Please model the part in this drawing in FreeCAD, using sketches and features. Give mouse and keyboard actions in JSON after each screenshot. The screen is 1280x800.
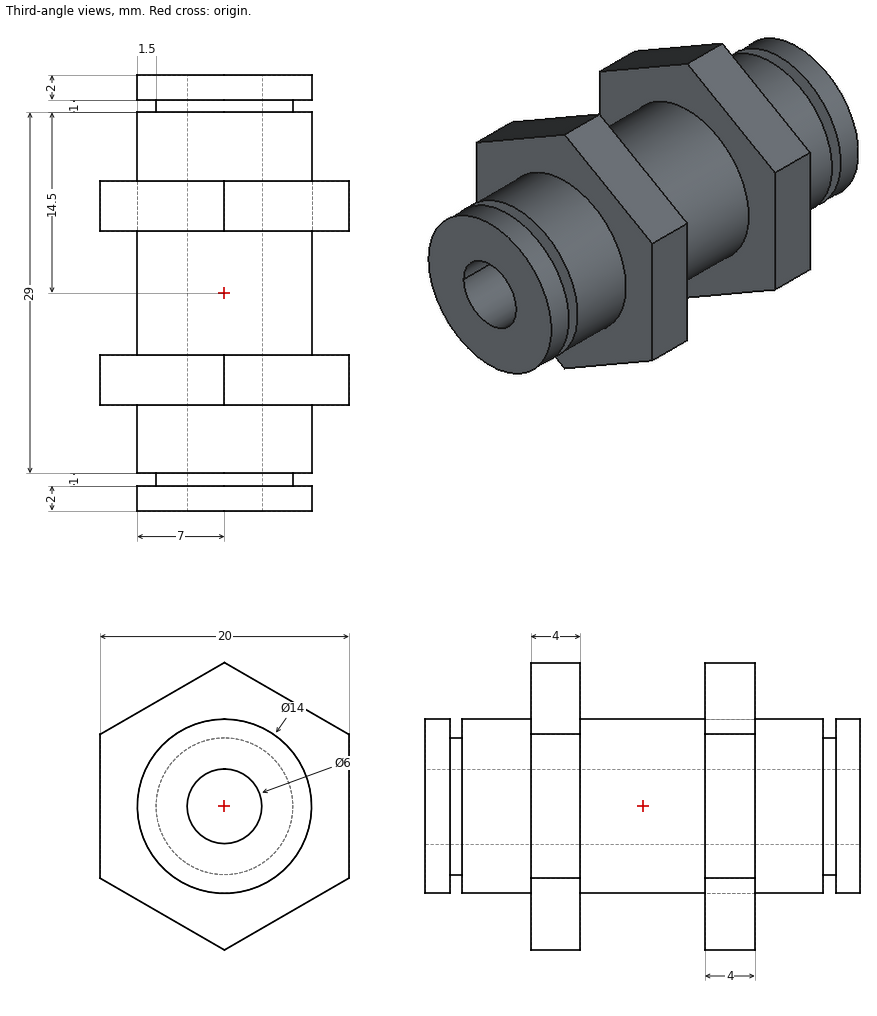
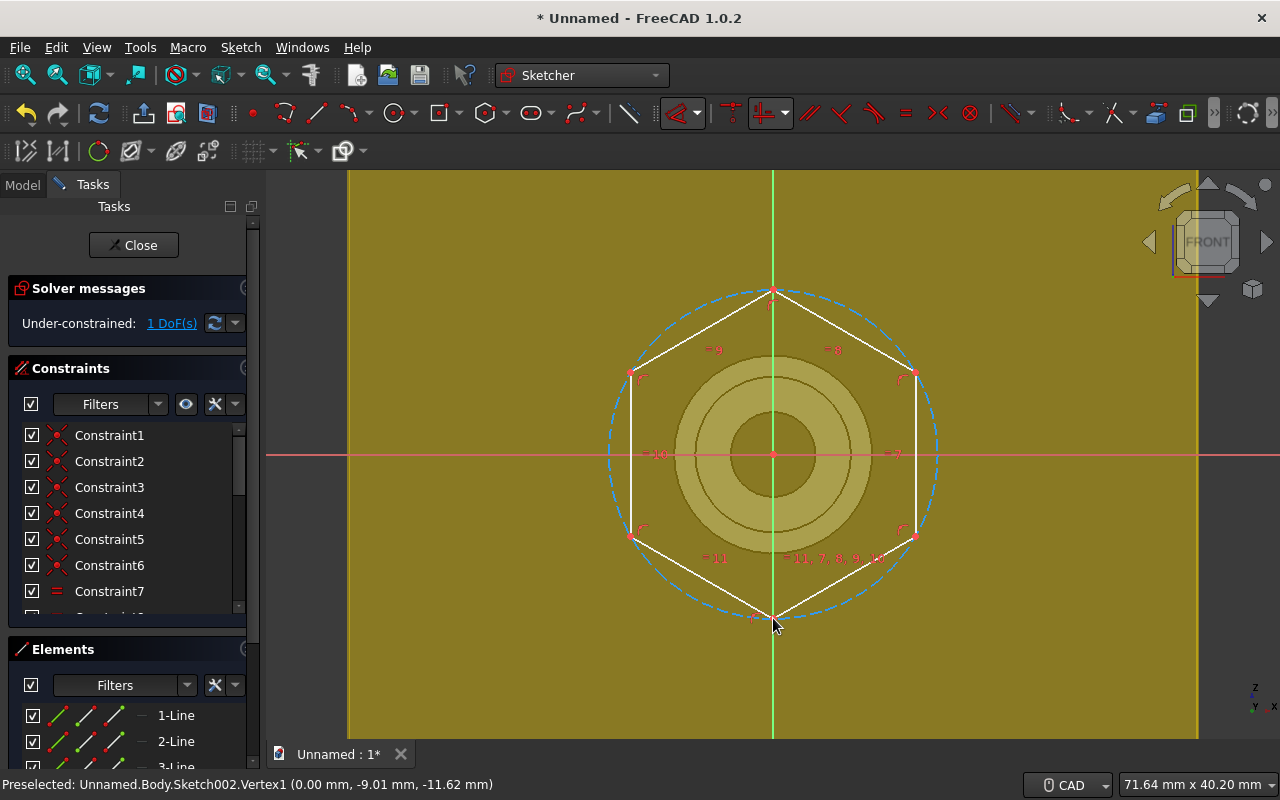
{"action": "left_click", "coordinate": [394, 114]}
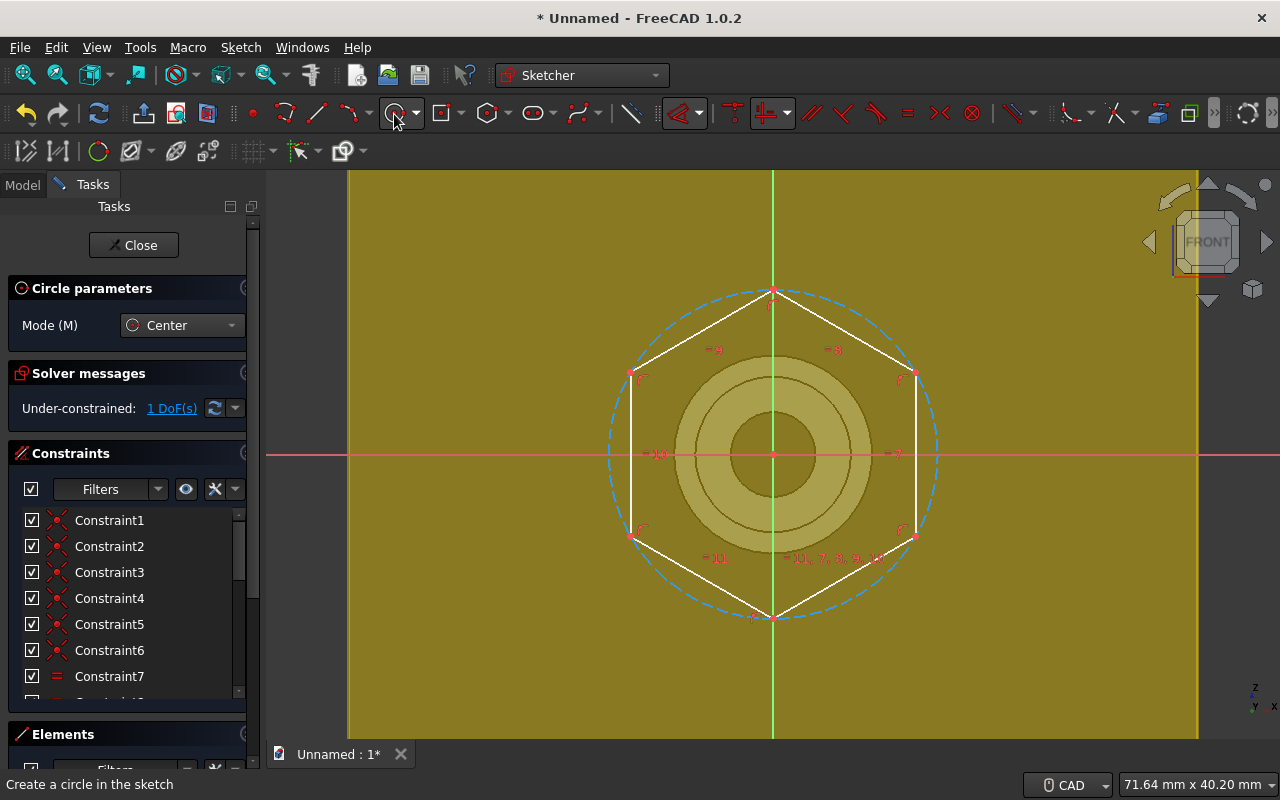
{"action": "left_click", "coordinate": [773, 455]}
{"action": "left_click", "coordinate": [843, 384]}
{"action": "key", "text": "Escape"}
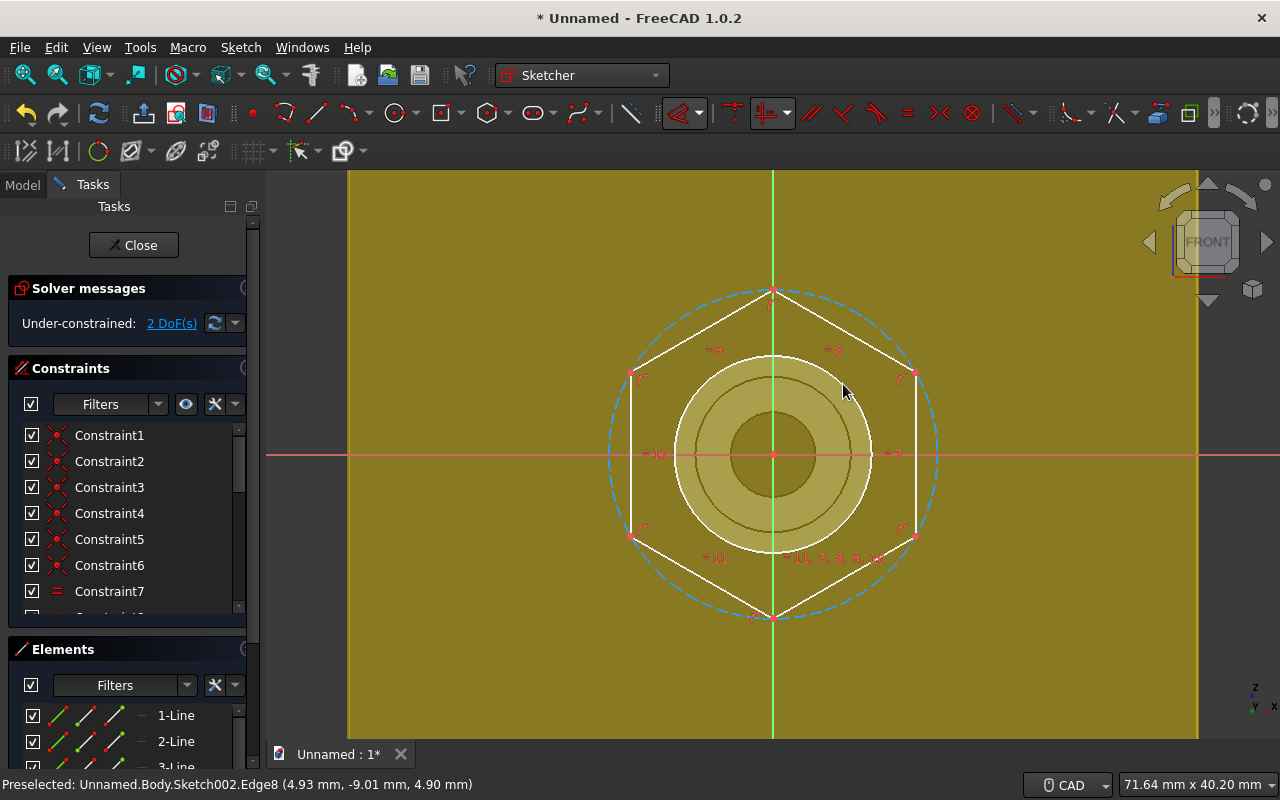
{"action": "left_click", "coordinate": [843, 385]}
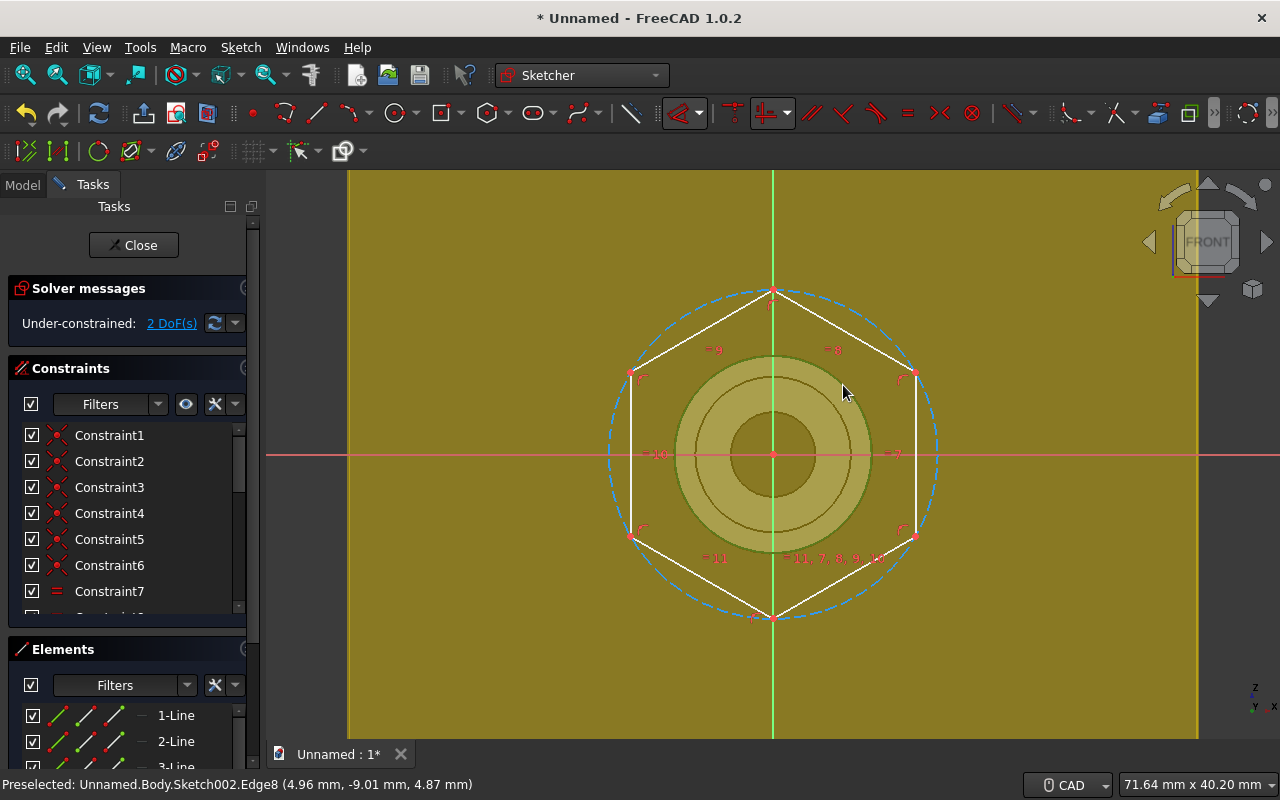
{"action": "left_click", "coordinate": [702, 114]}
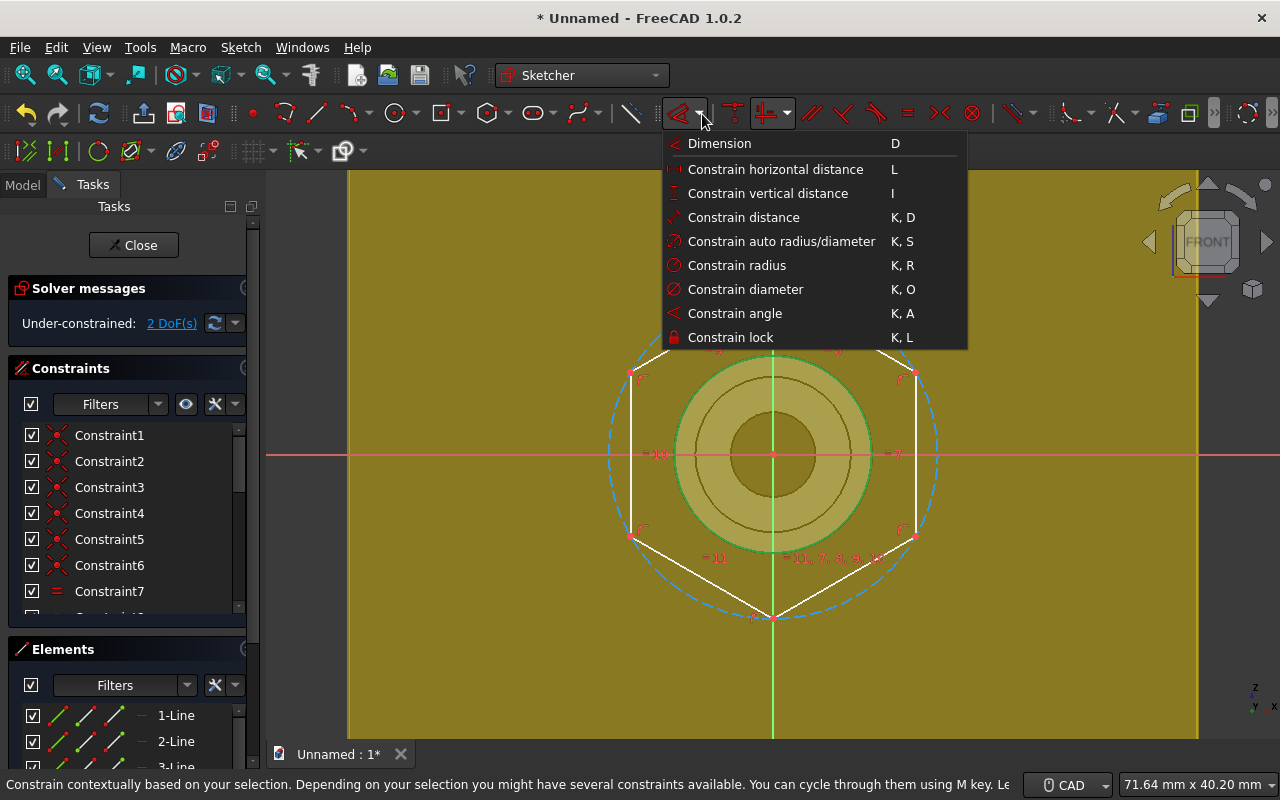
{"action": "left_click", "coordinate": [815, 289]}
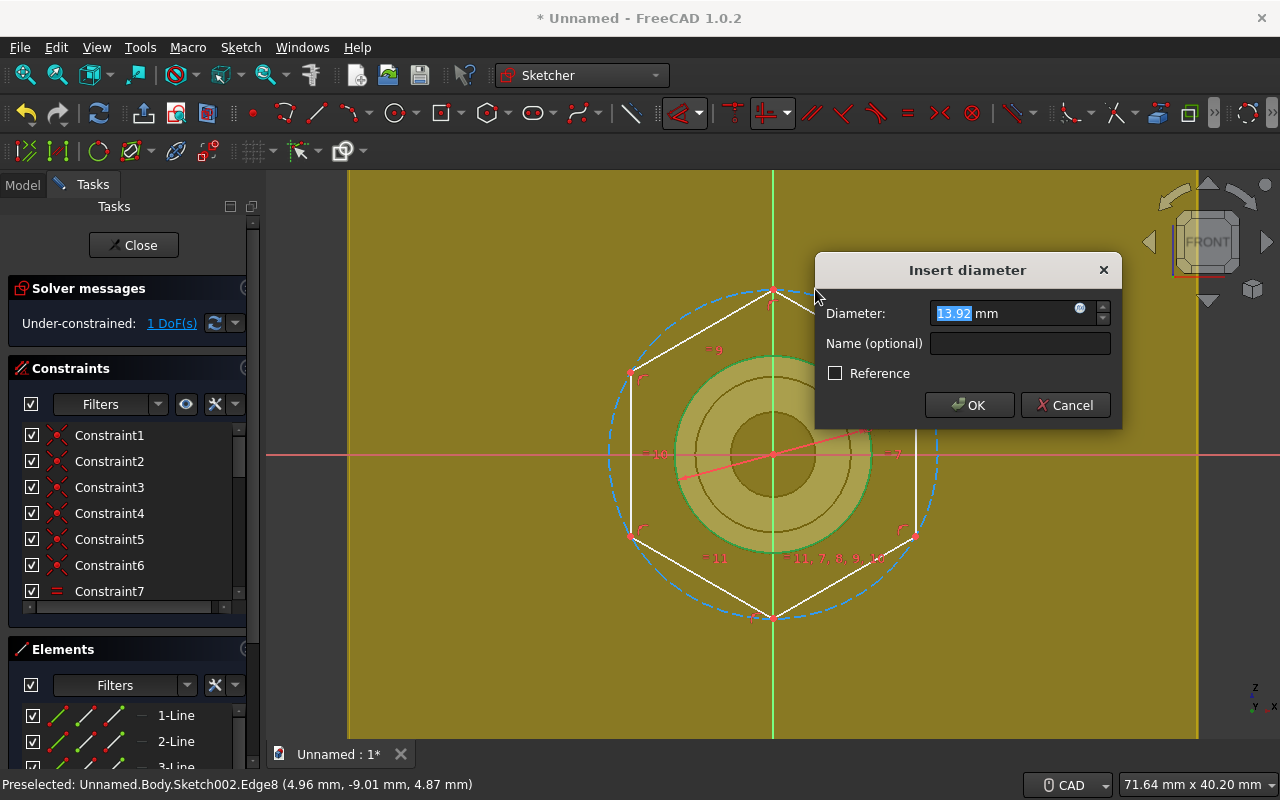
{"action": "type", "text": "14"}
{"action": "key", "text": "Return"}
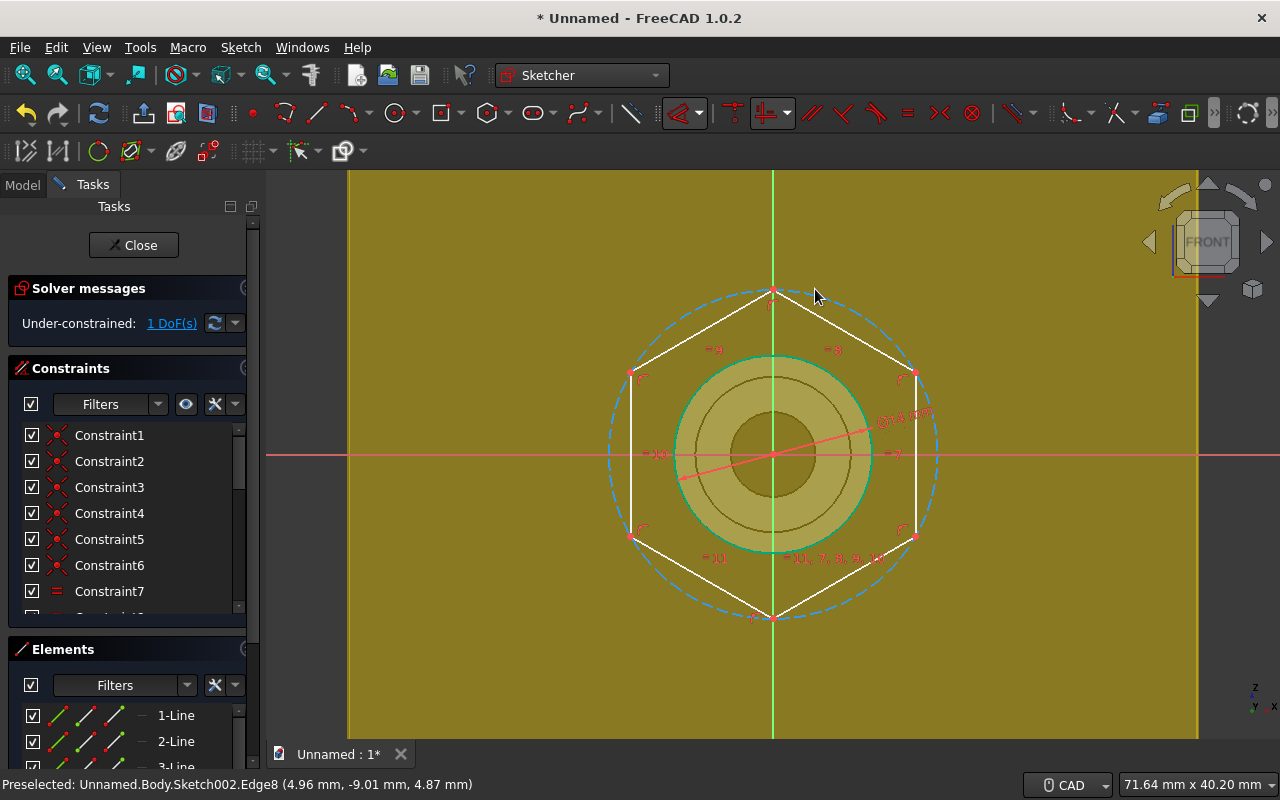
{"action": "left_click", "coordinate": [631, 372]}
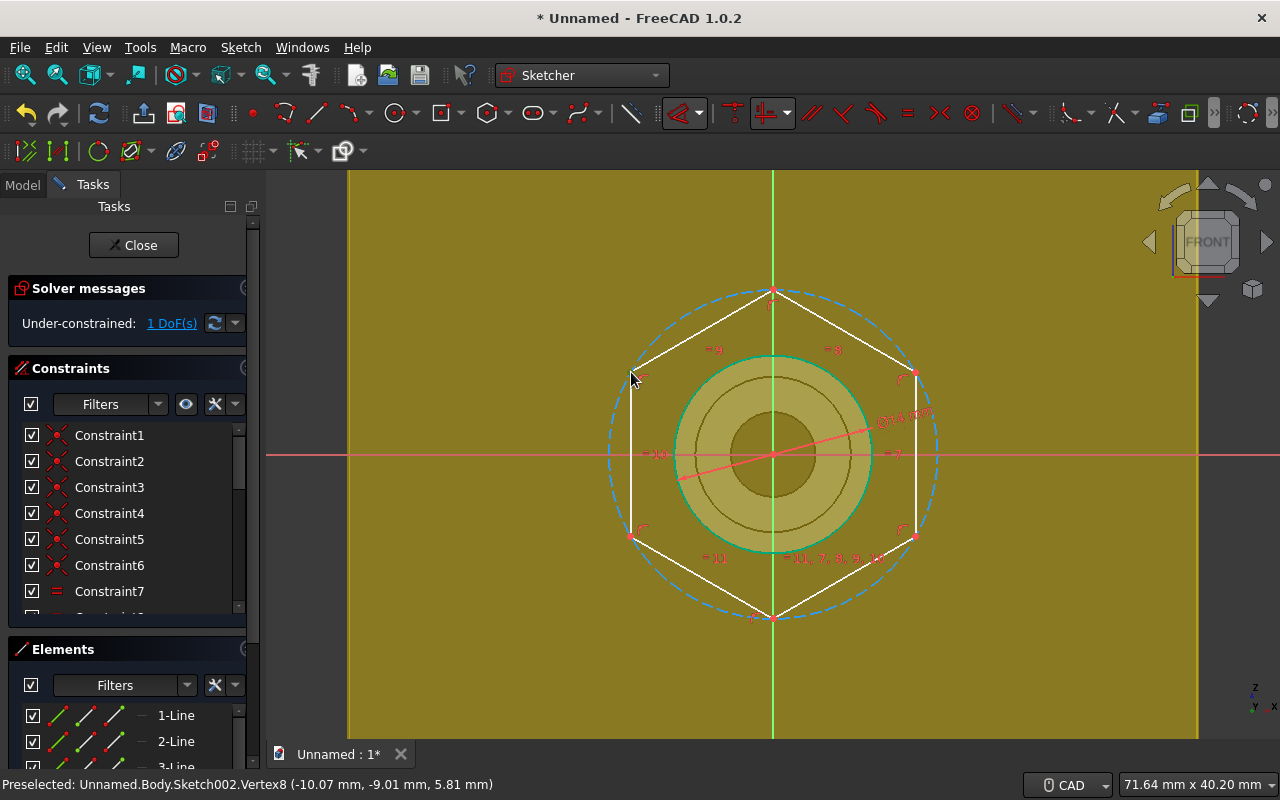
{"action": "left_click", "coordinate": [916, 537]}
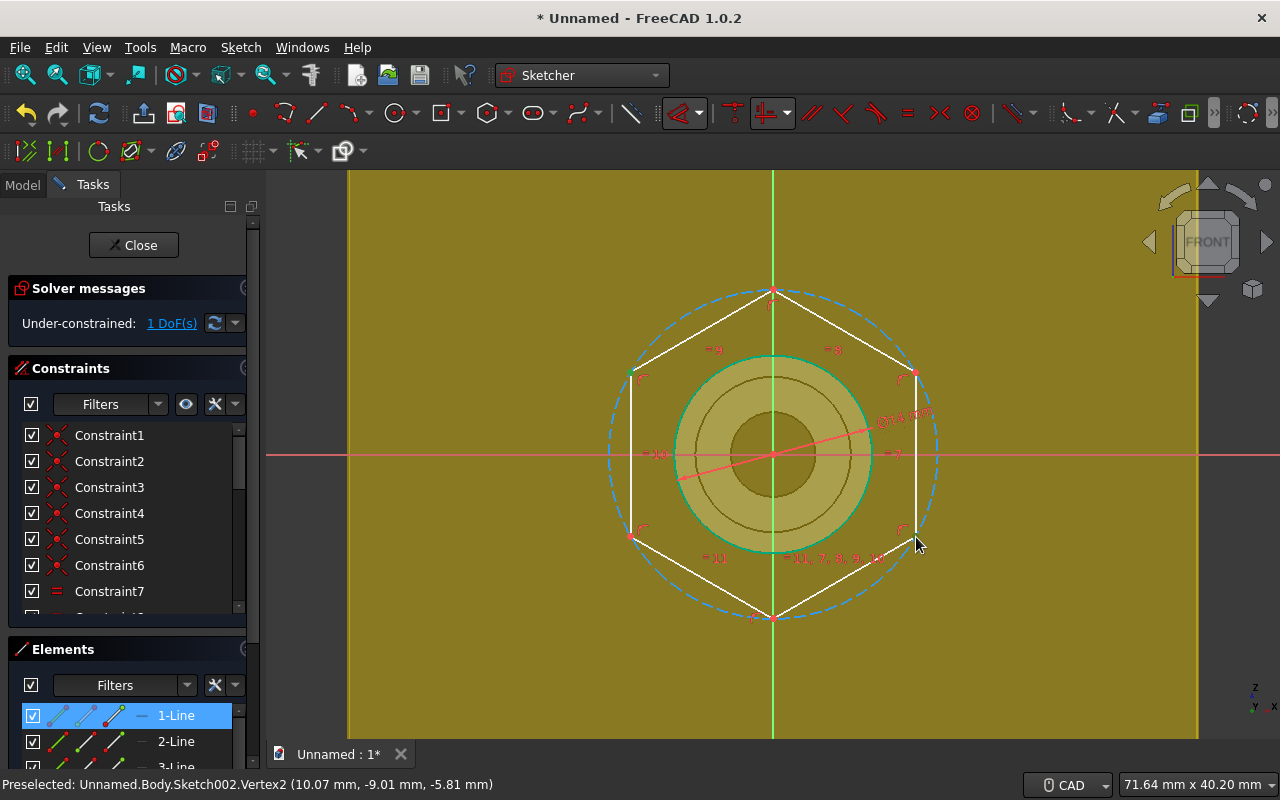
{"action": "key", "text": "l"}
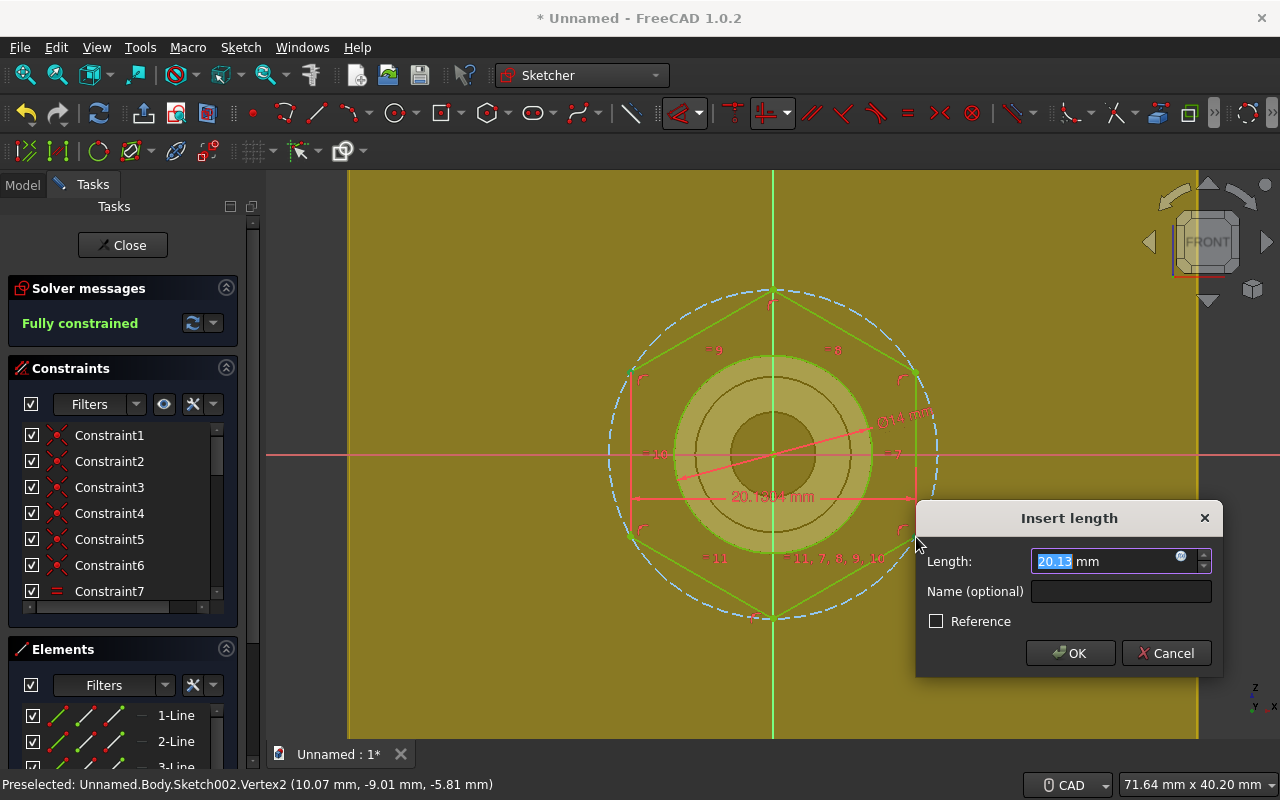
{"action": "type", "text": "20"}
{"action": "key", "text": "Return"}